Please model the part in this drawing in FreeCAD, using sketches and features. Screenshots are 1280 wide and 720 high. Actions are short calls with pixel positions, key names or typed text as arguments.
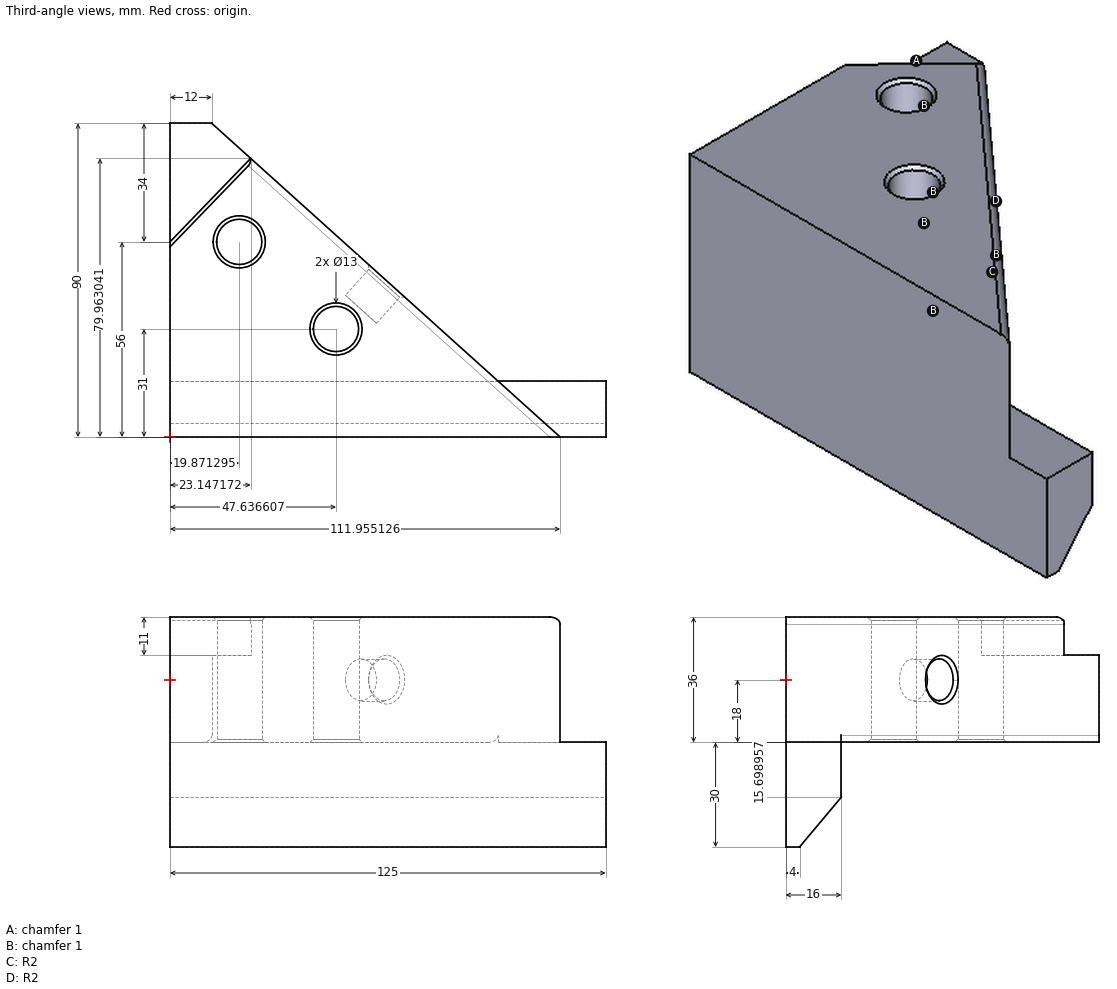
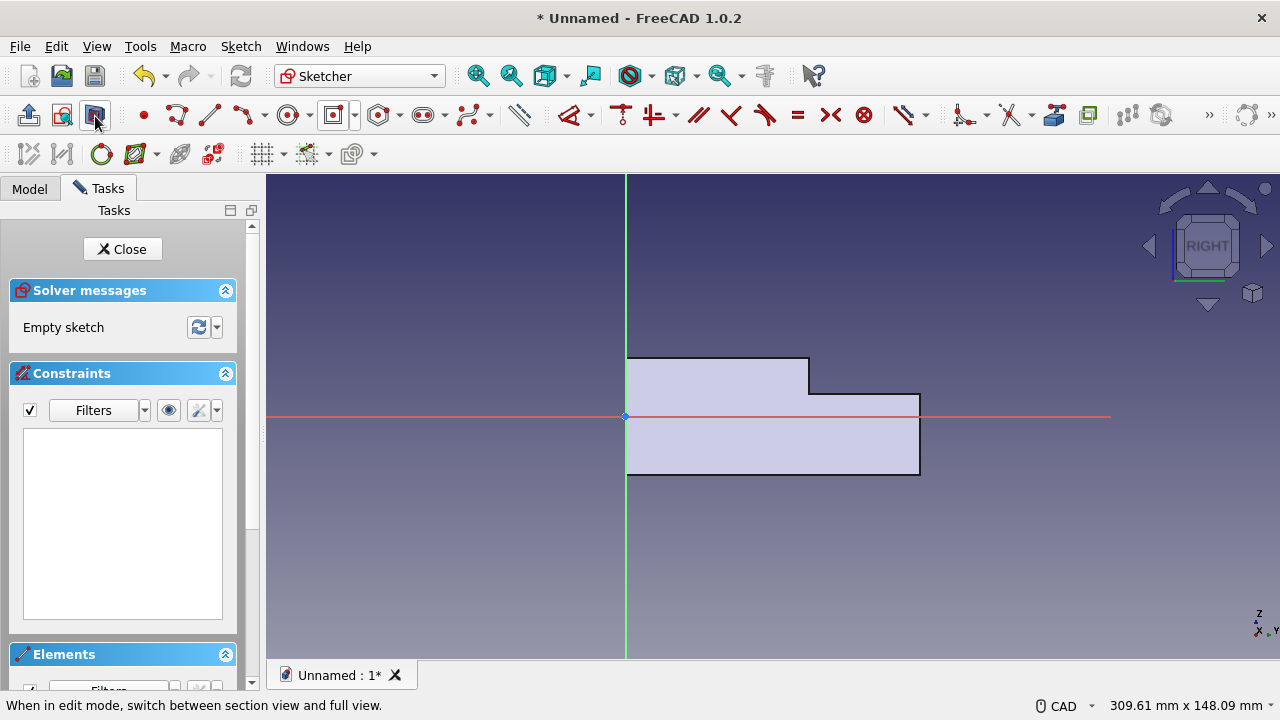
scroll(588, 591, up, 3)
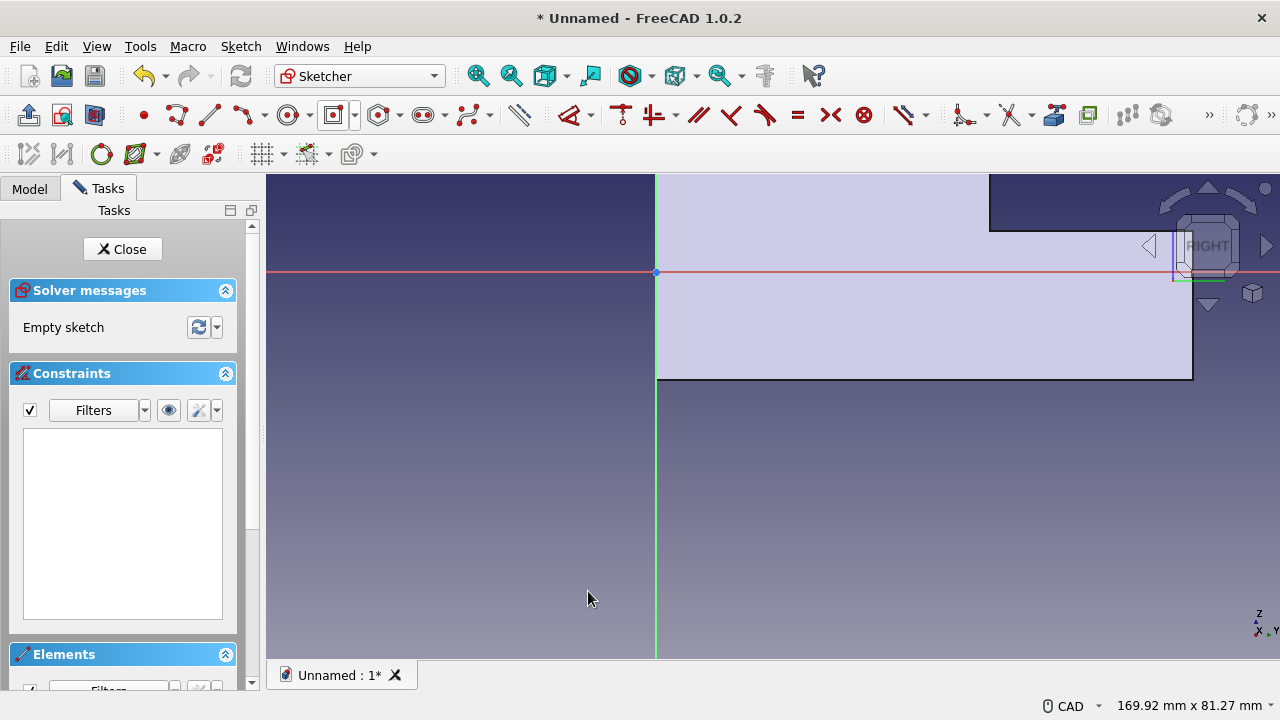
click(177, 116)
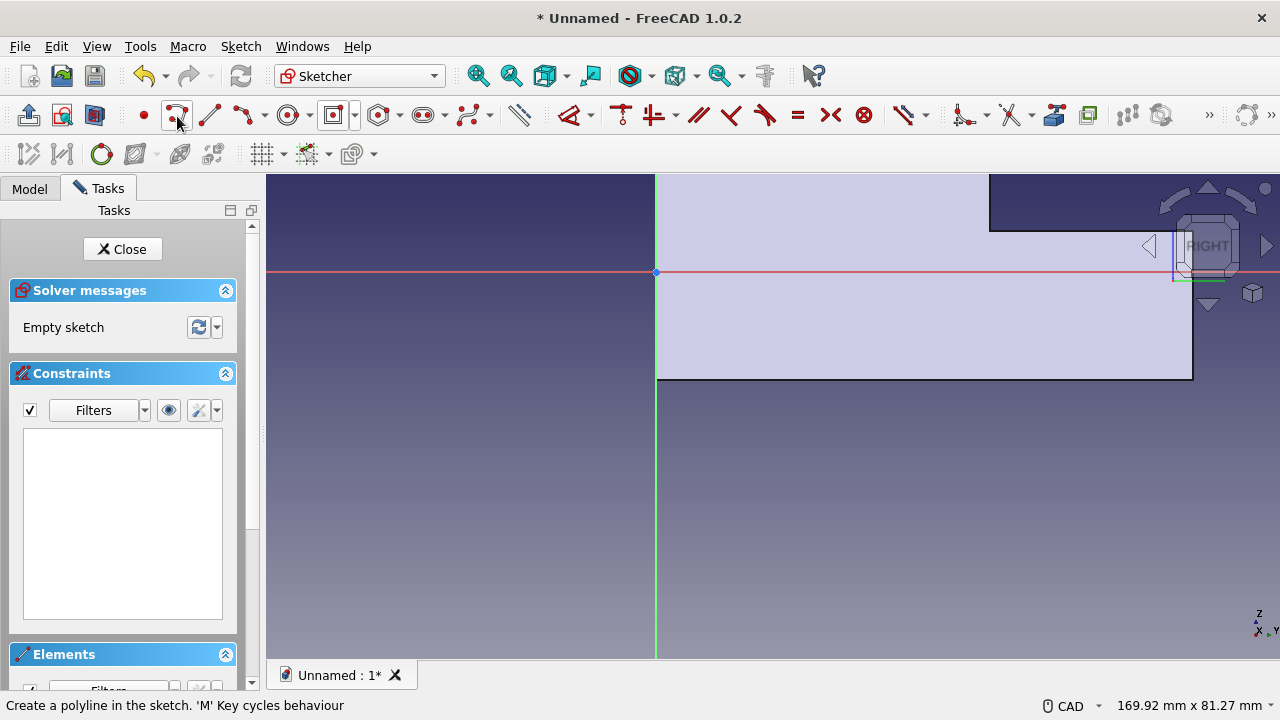
click(656, 380)
click(752, 380)
click(752, 473)
click(680, 559)
click(665, 559)
click(656, 381)
key(Escape)
key(Escape)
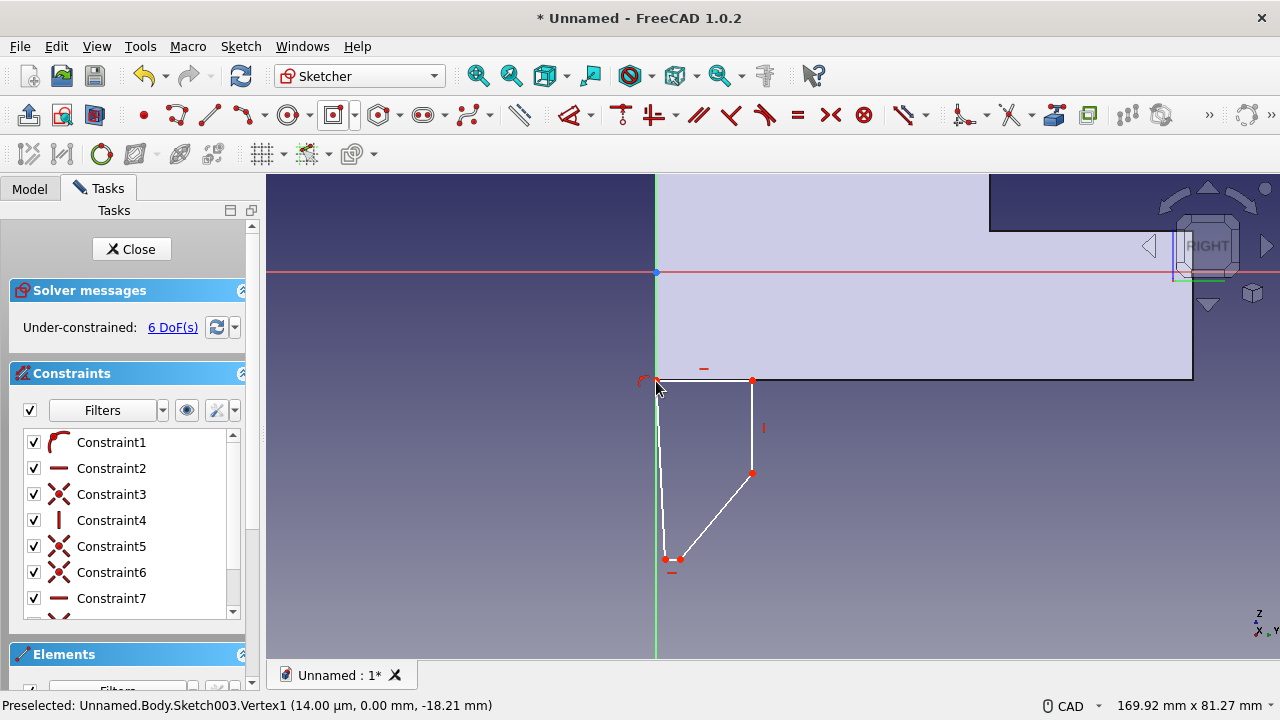
click(659, 435)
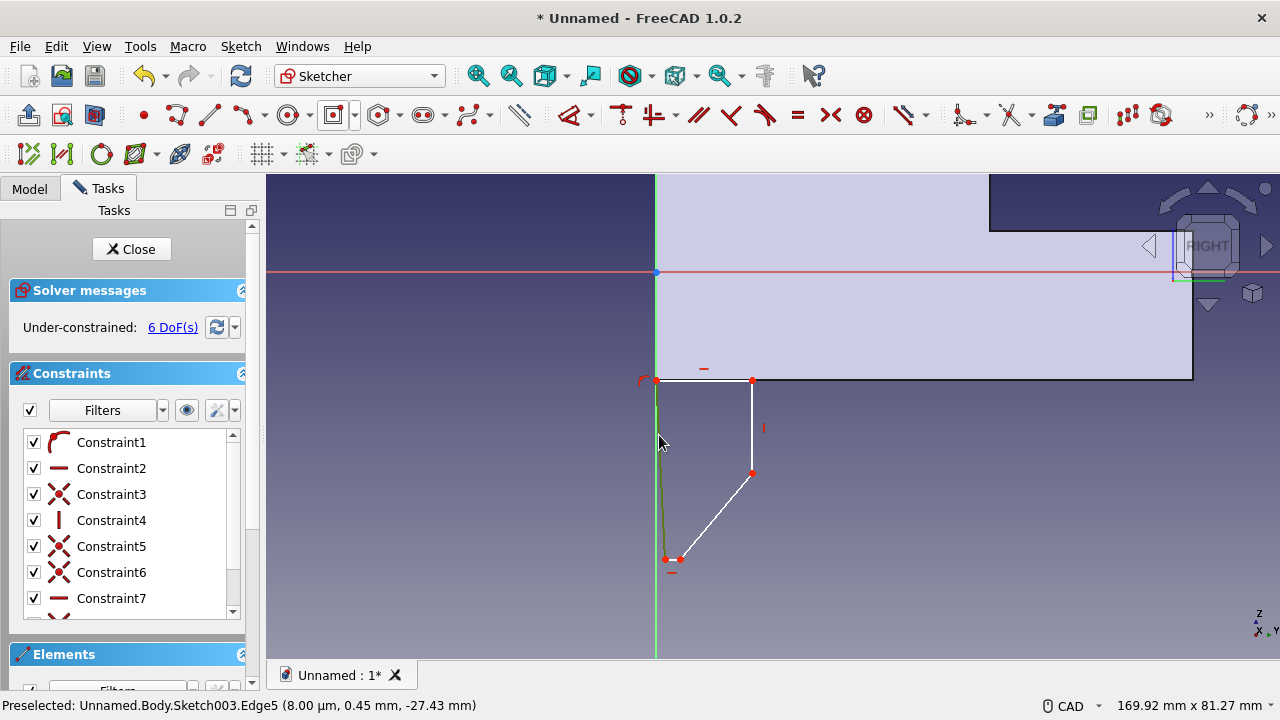
key(v)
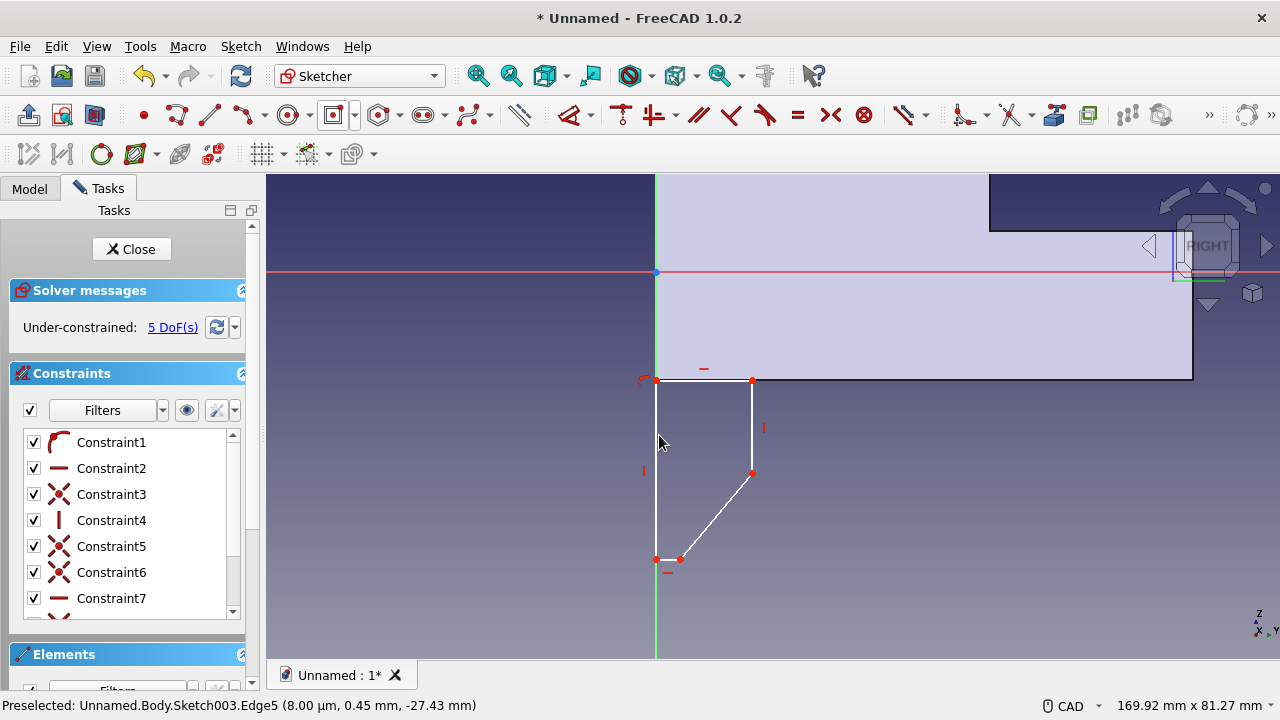
click(568, 116)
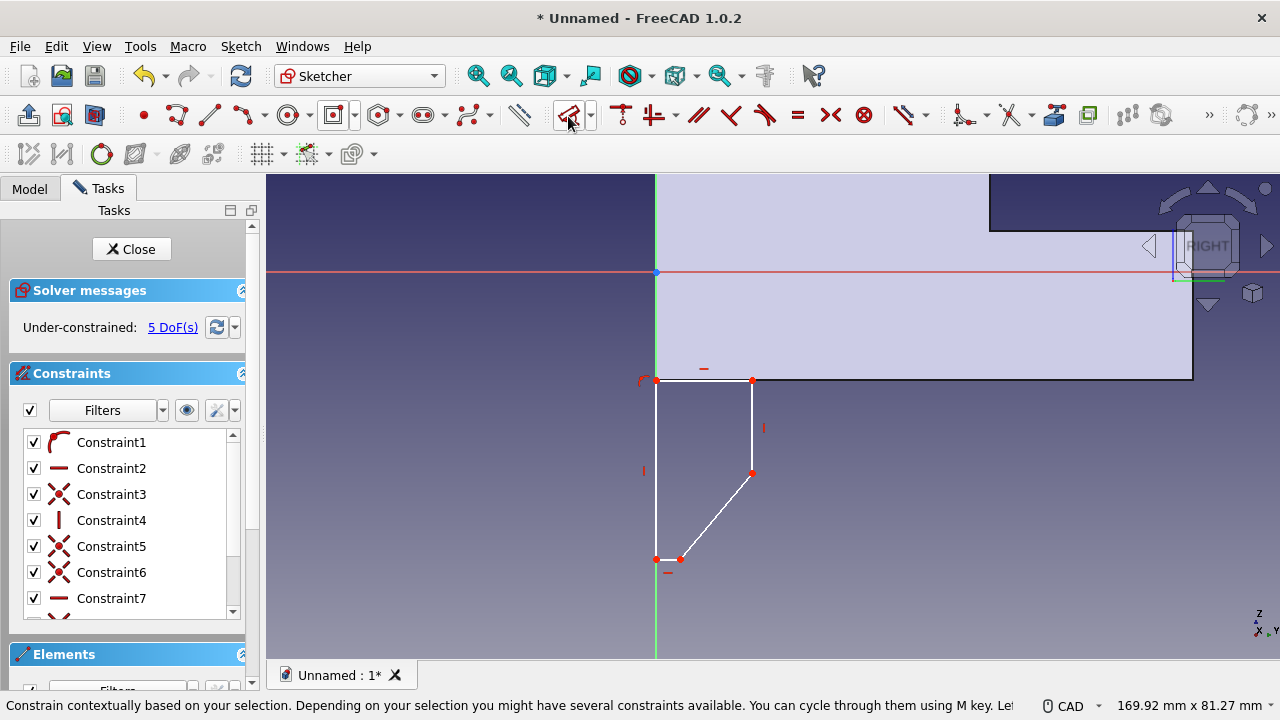
scroll(671, 560, up, 3)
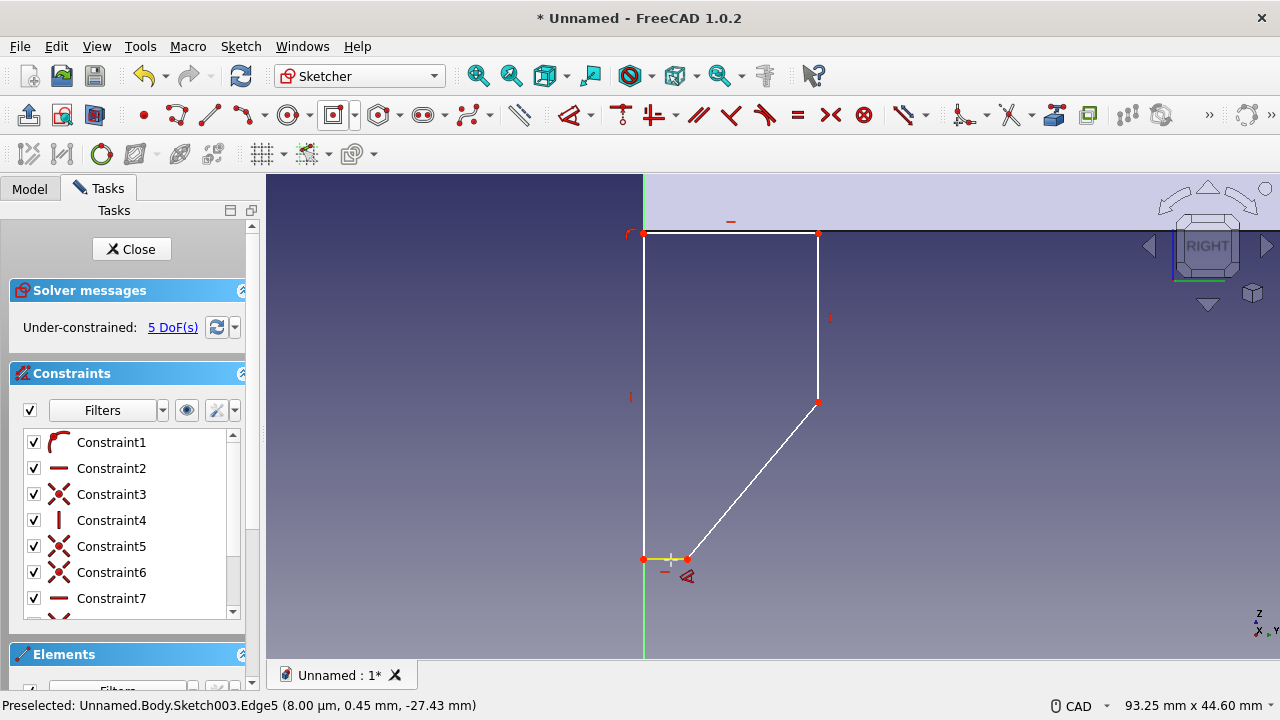
click(670, 559)
click(665, 593)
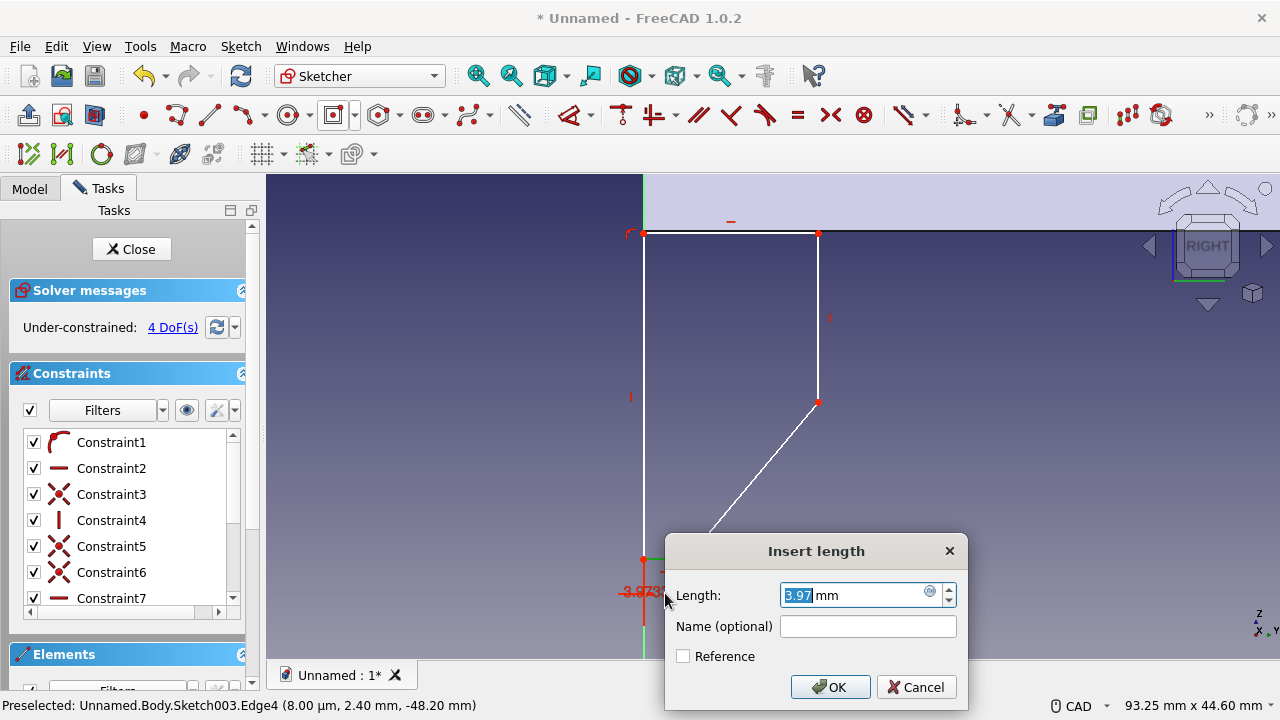
text(4)
key(Return)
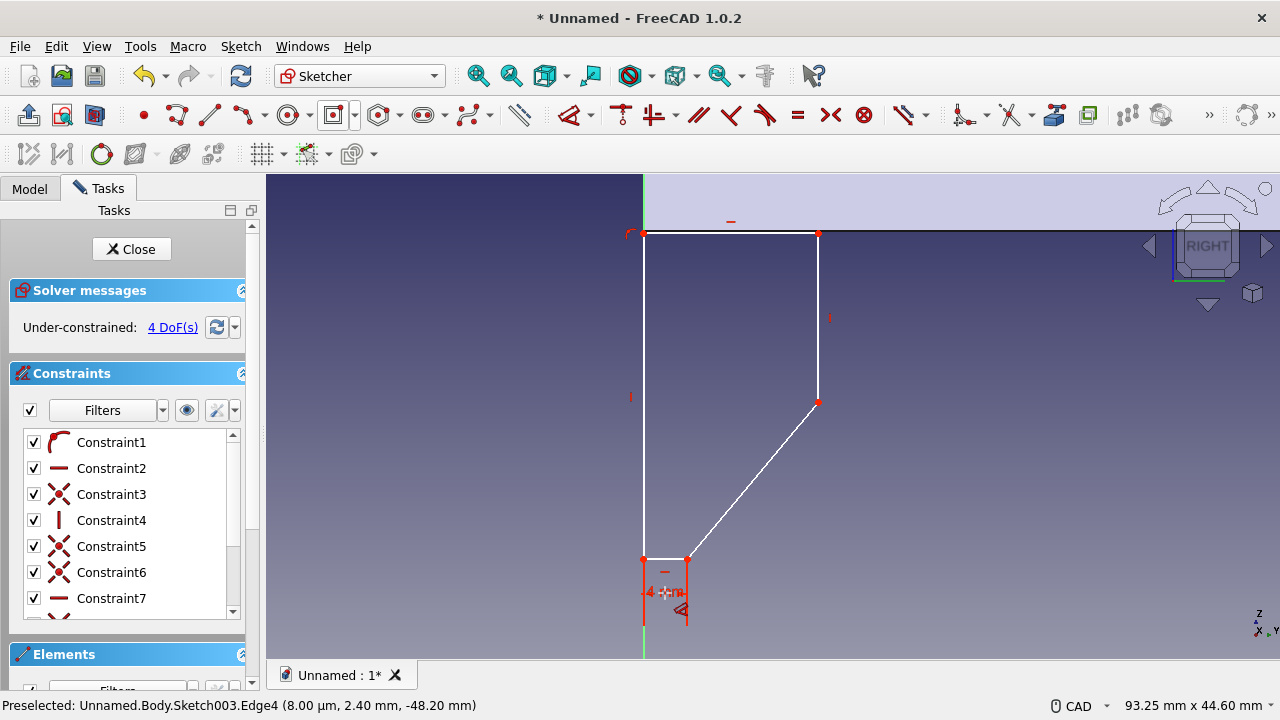
click(696, 233)
click(731, 267)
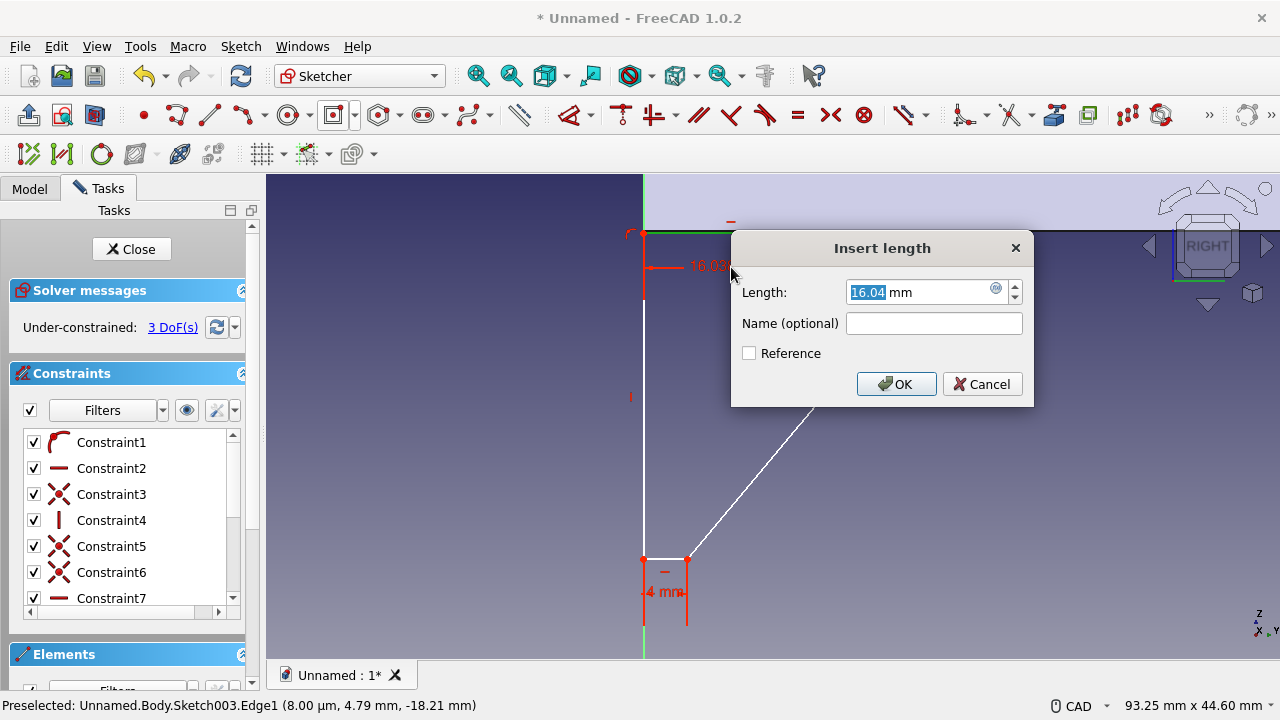
text(16)
key(Return)